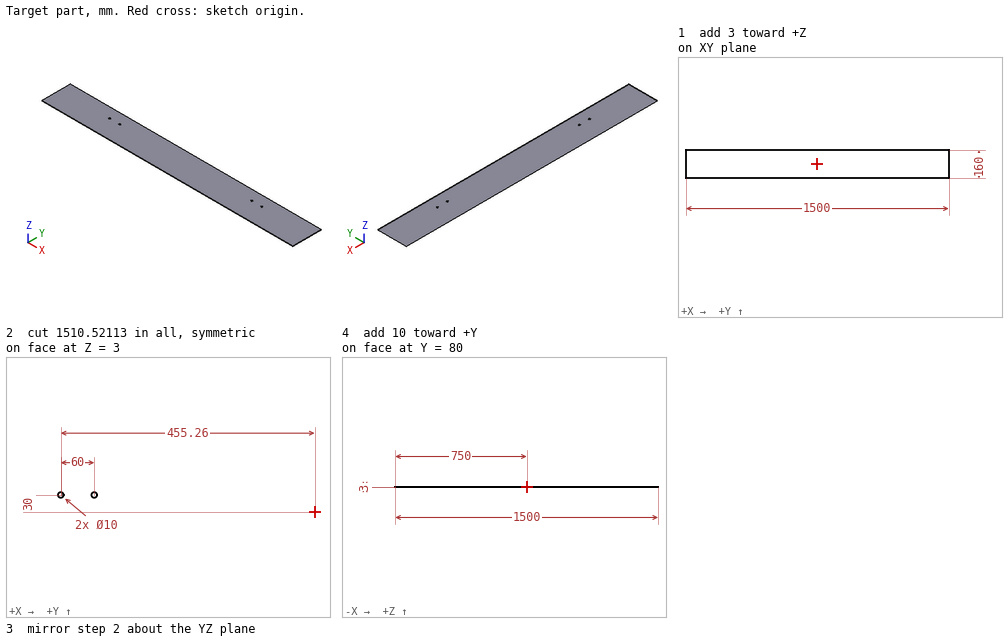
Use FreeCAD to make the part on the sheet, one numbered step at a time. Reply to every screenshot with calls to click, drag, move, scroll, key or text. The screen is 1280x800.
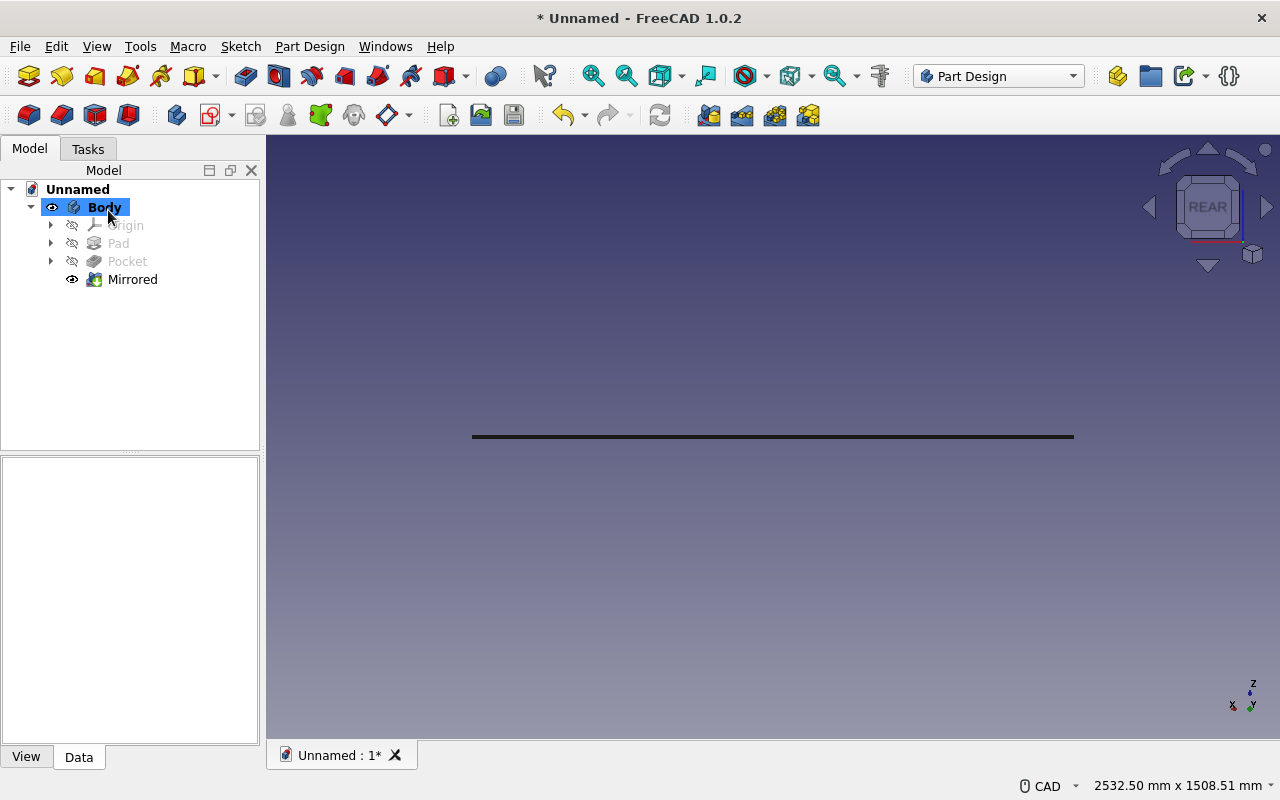
scroll(516, 436, up, 15)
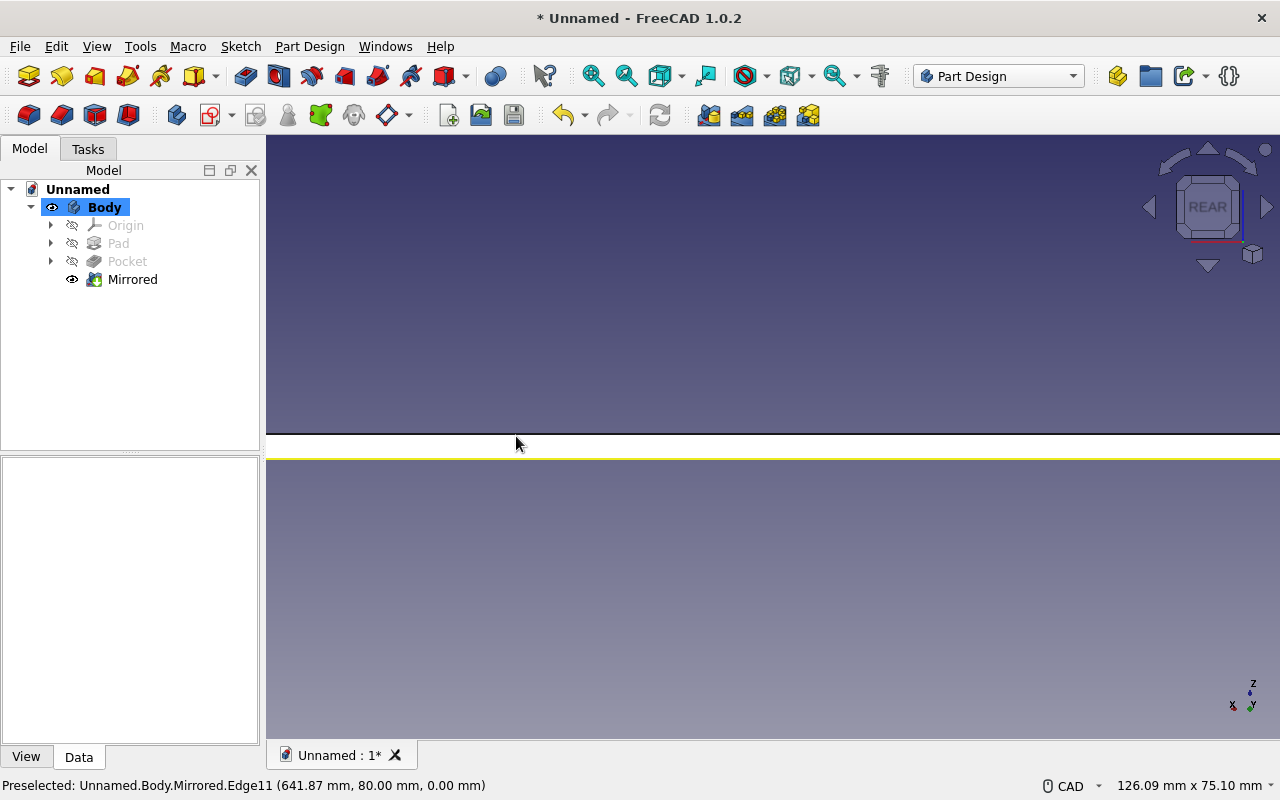
click(503, 446)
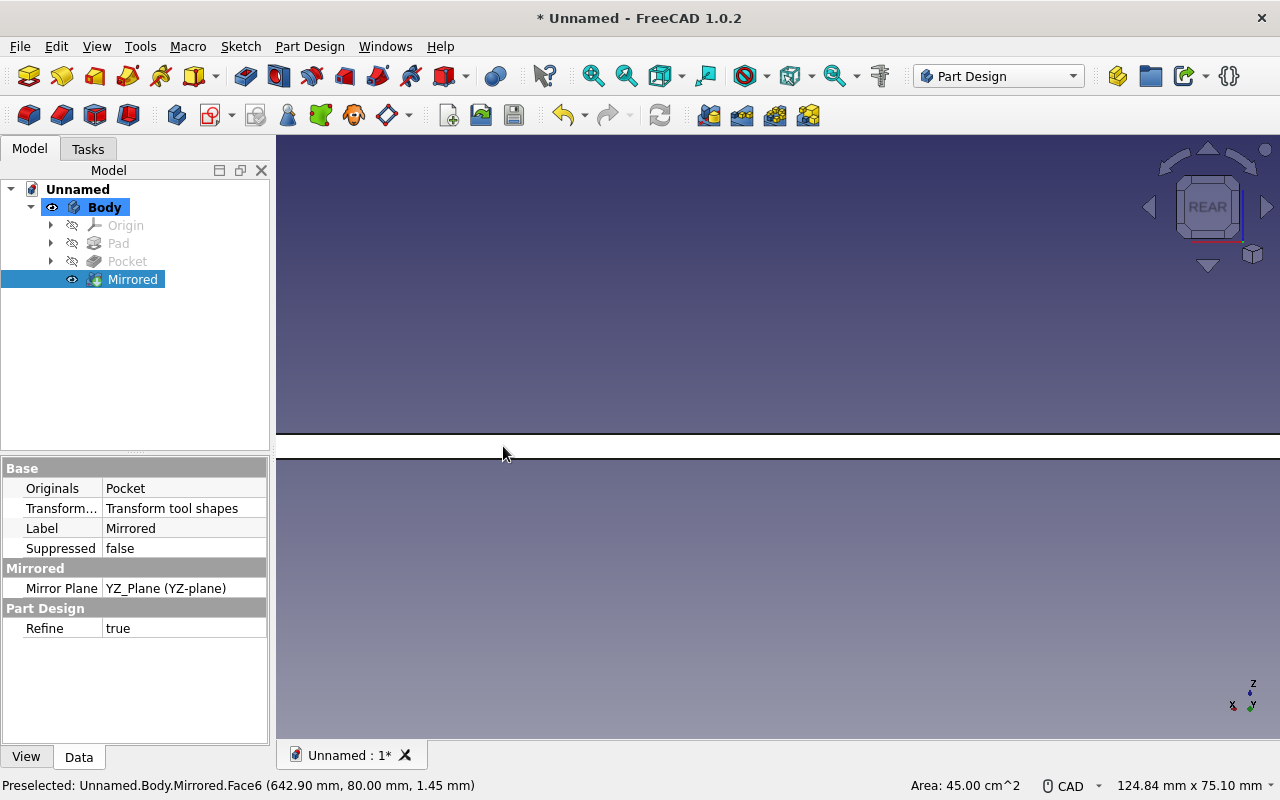
click(210, 116)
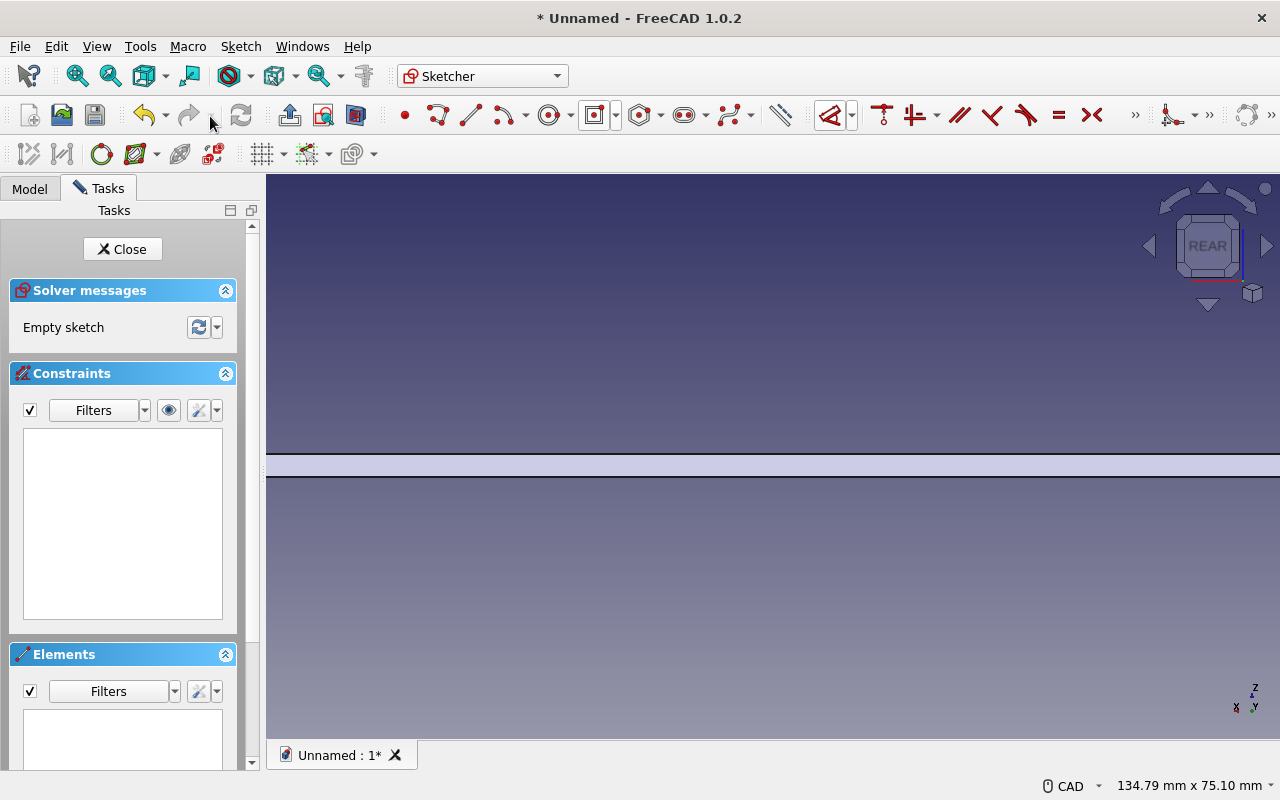
scroll(461, 456, down, 15)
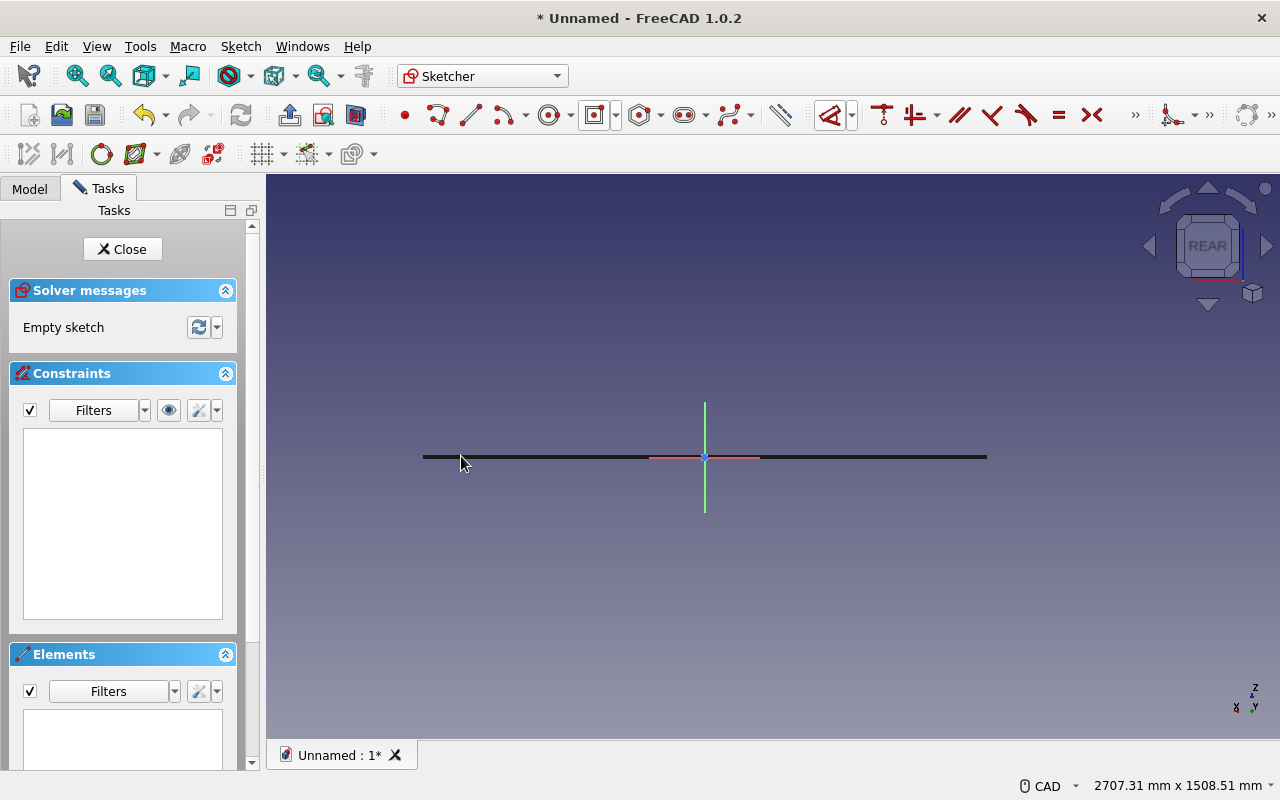
key(g)
key(r)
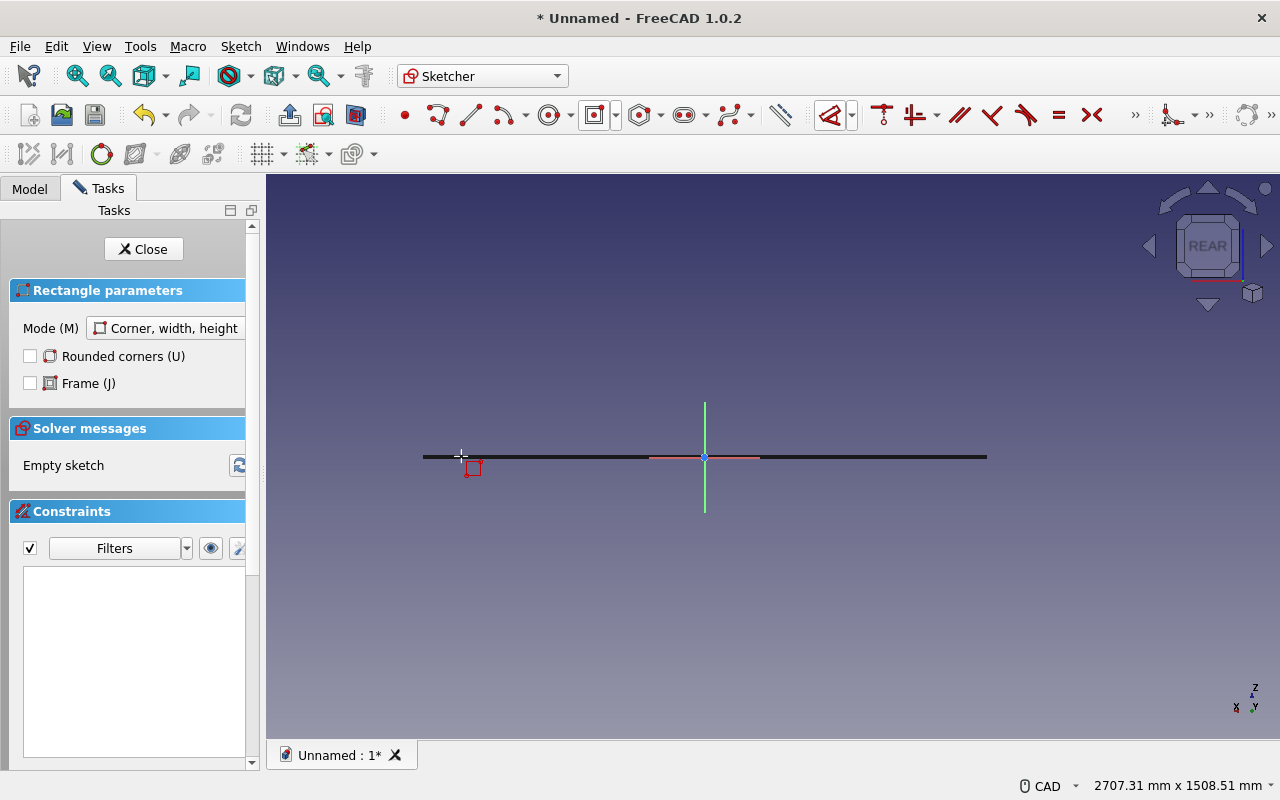
scroll(424, 456, up, 14)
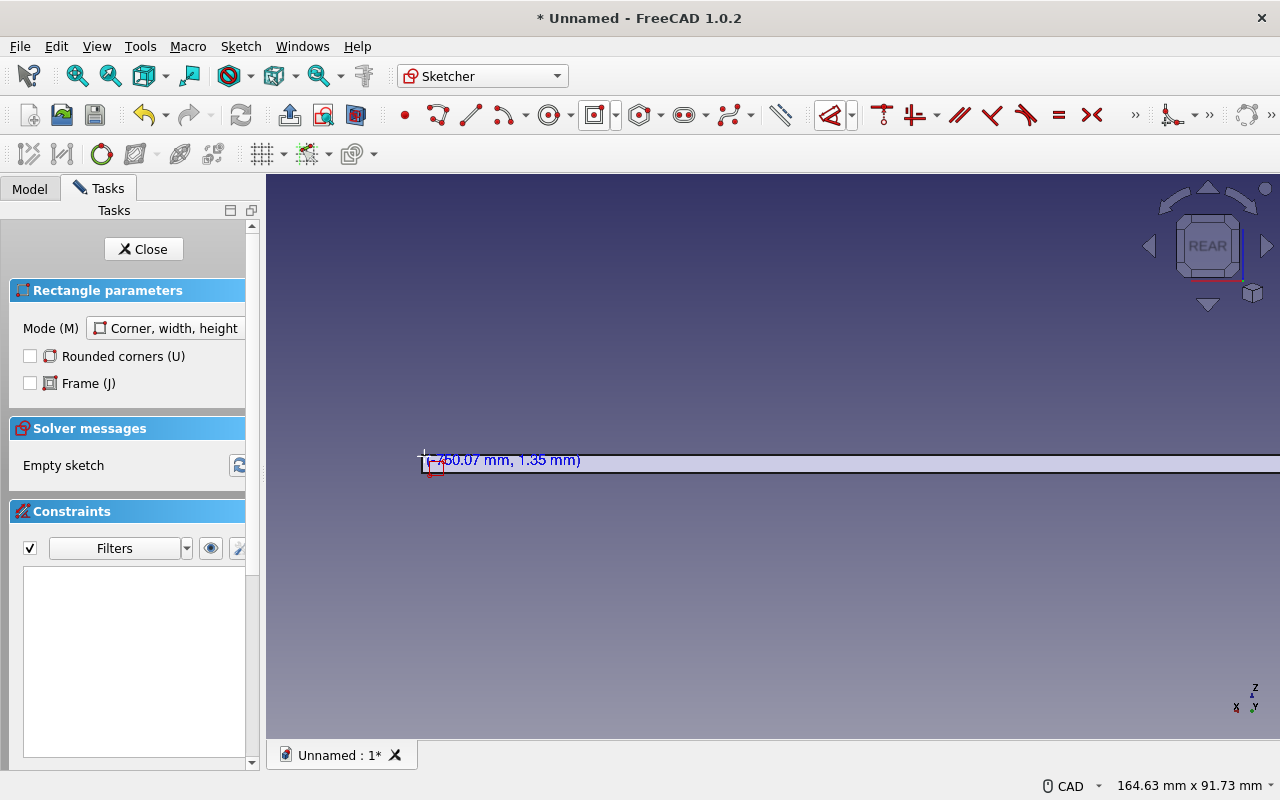
click(422, 455)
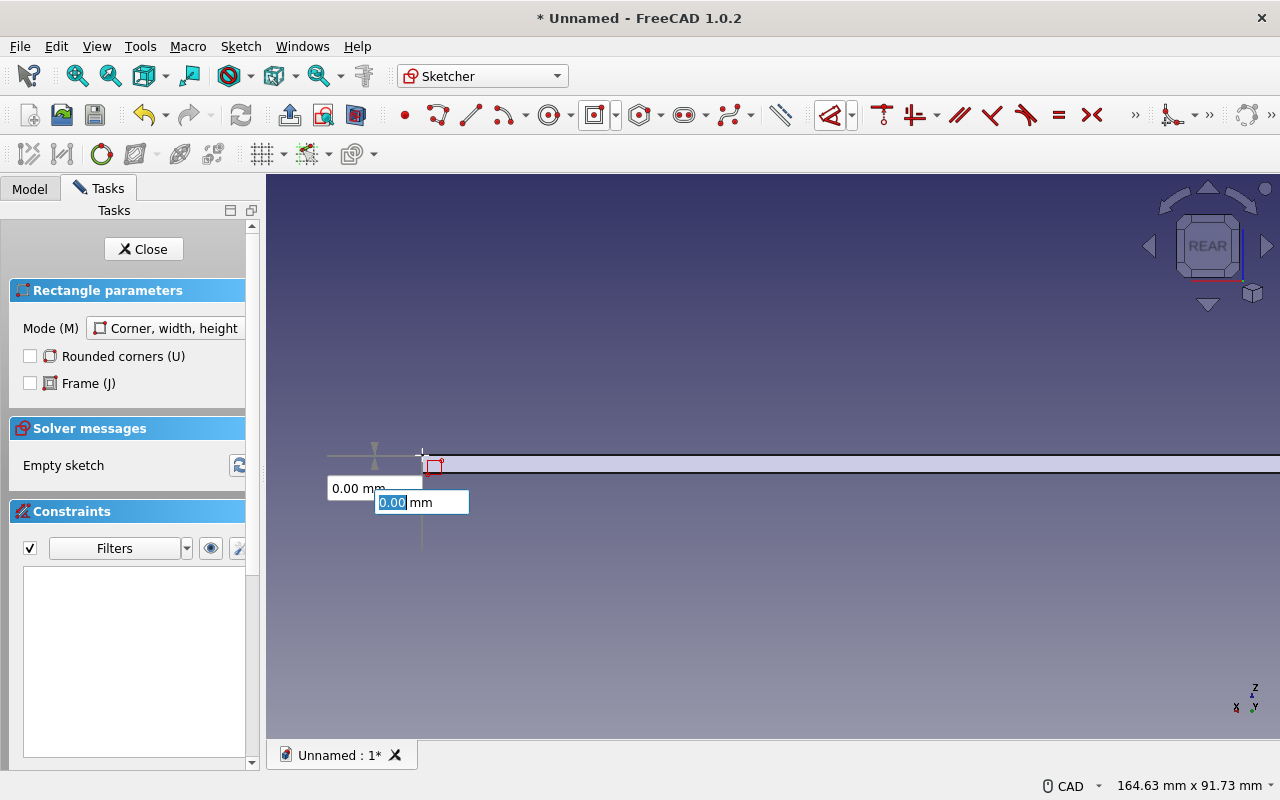
scroll(424, 456, down, 14)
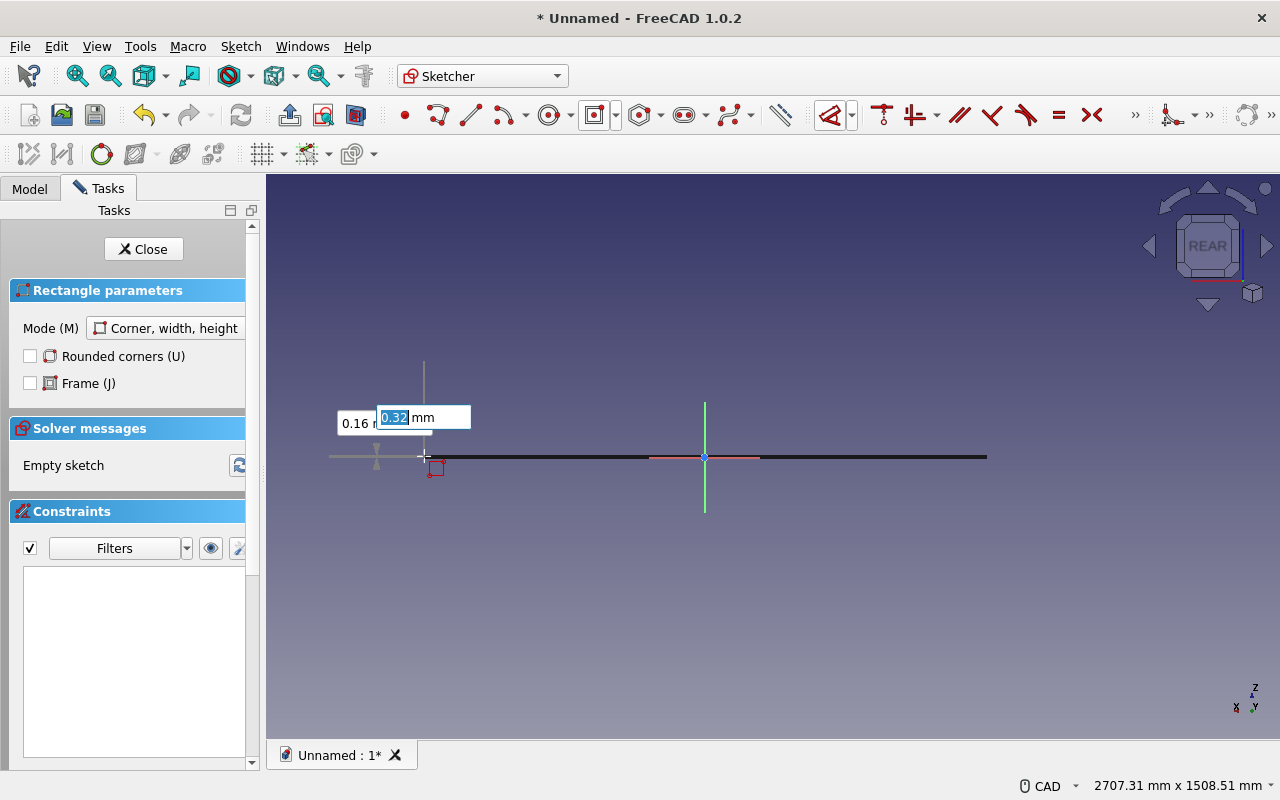
click(986, 458)
key(Escape)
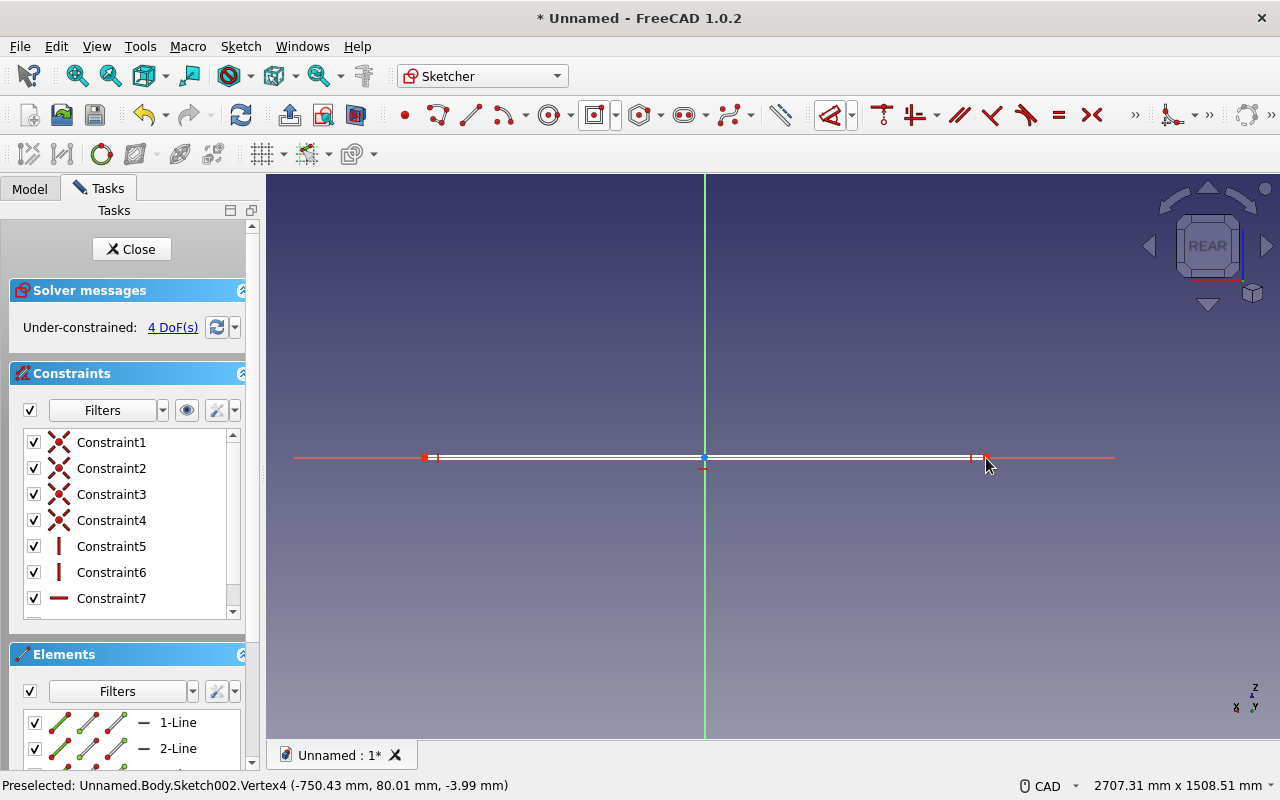
scroll(424, 459, up, 8)